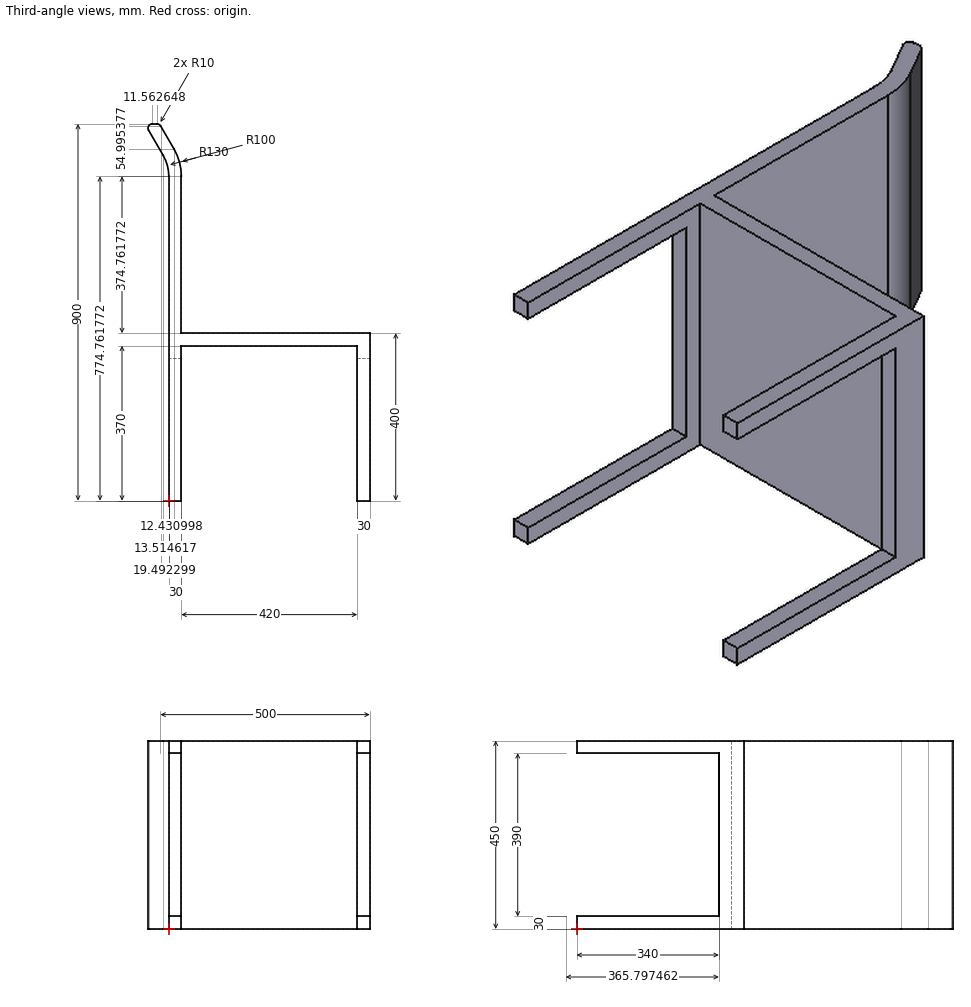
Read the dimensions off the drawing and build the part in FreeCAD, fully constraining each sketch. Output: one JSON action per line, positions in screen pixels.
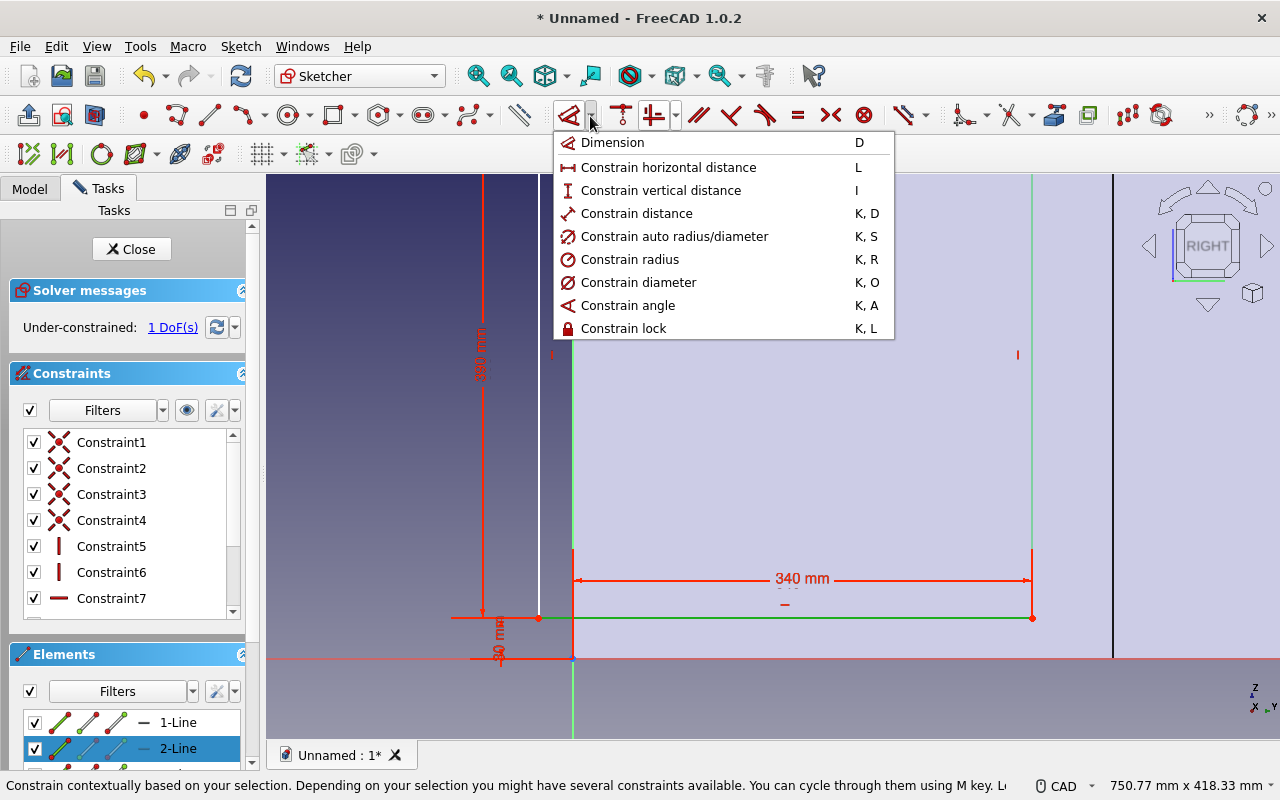
{"action": "left_click", "coordinate": [724, 168]}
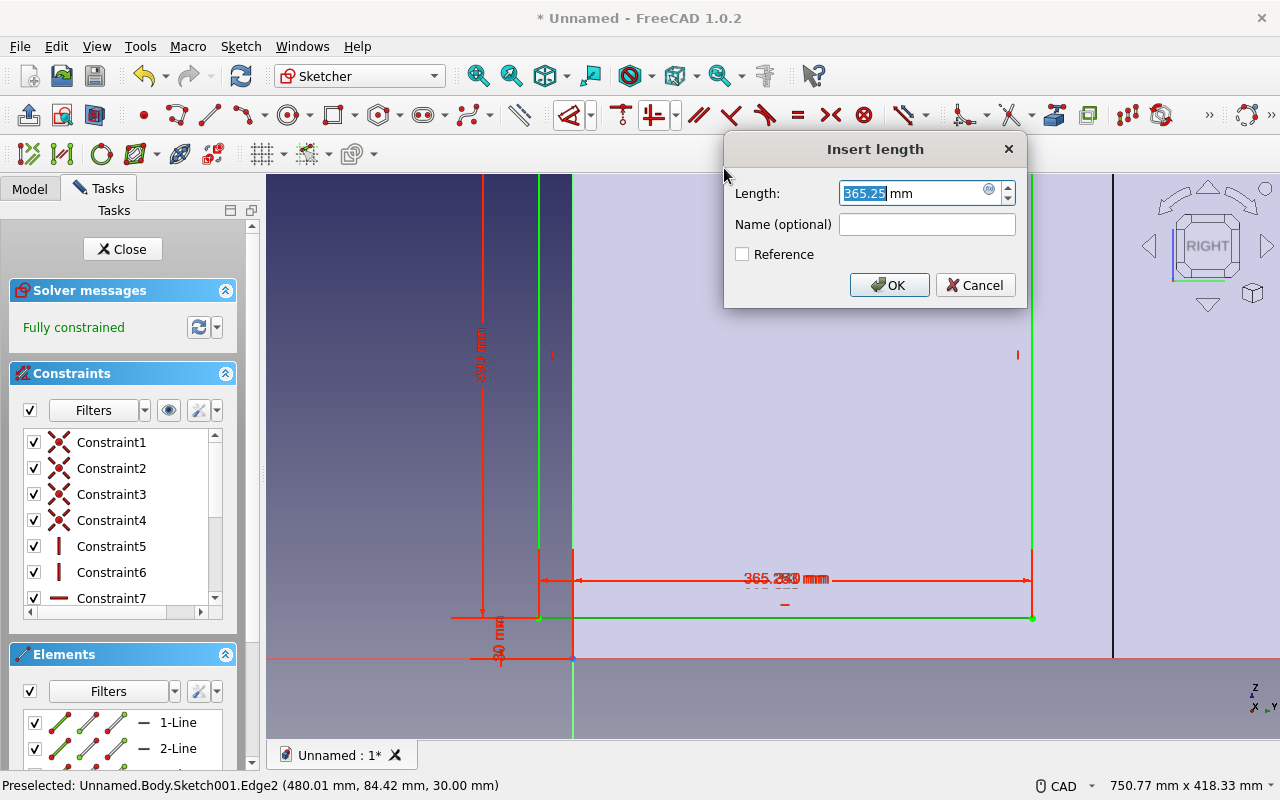
{"action": "type", "text": "365.797462"}
{"action": "key", "text": "Return"}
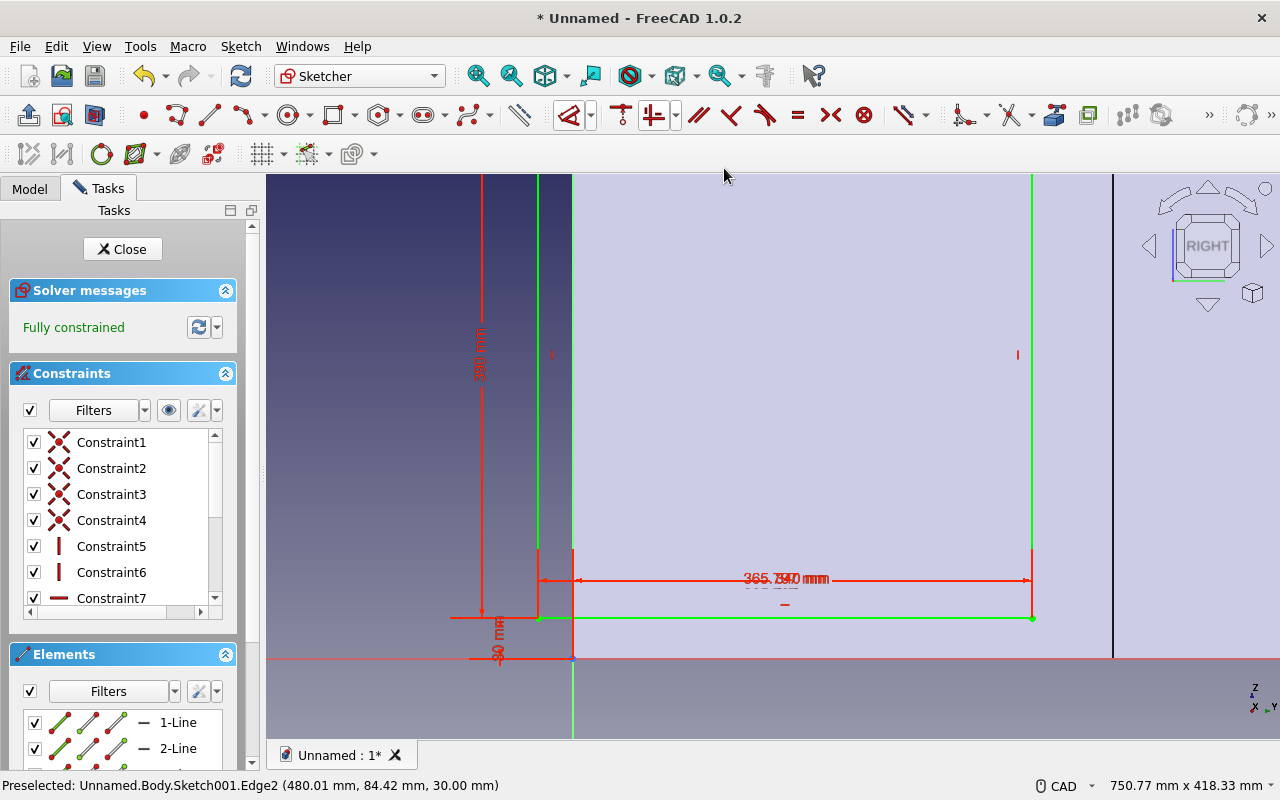
{"action": "left_click", "coordinate": [123, 249]}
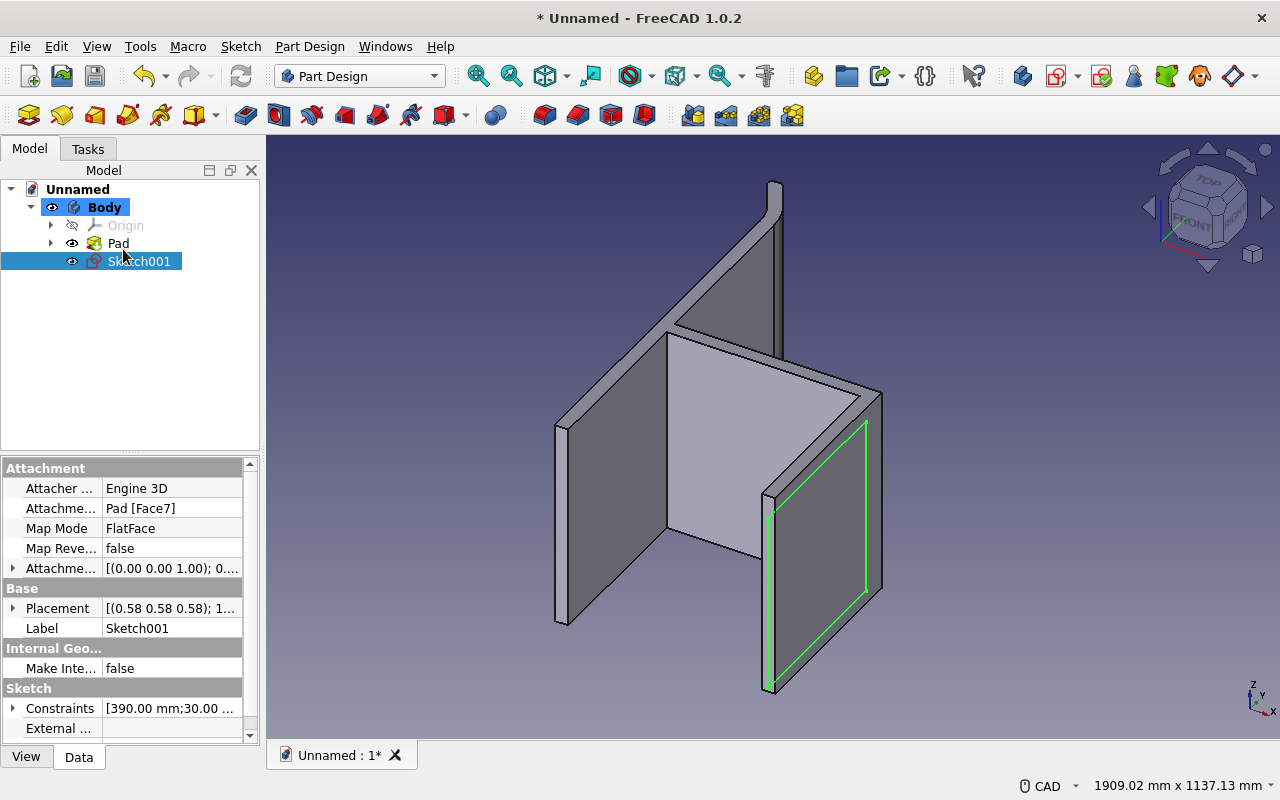
{"action": "left_click", "coordinate": [246, 116]}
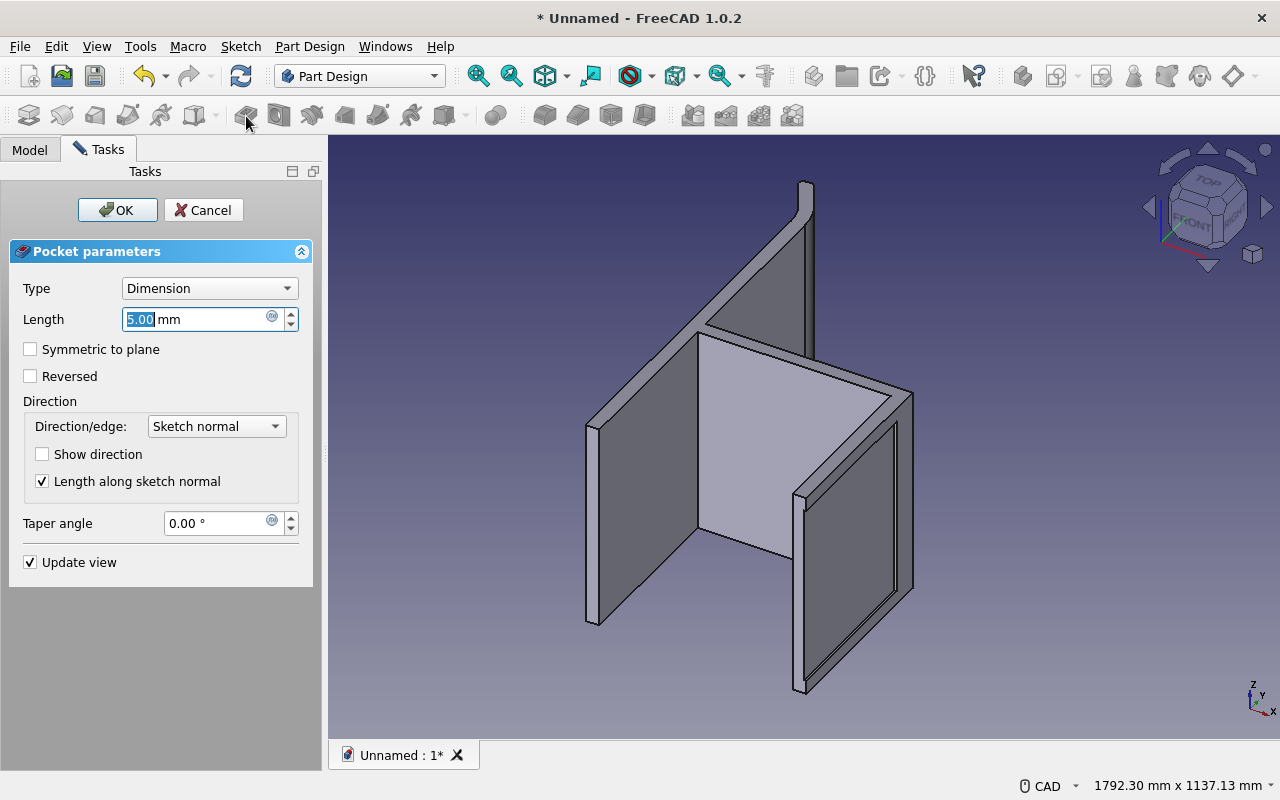
{"action": "type", "text": "500"}
{"action": "key", "text": "Tab"}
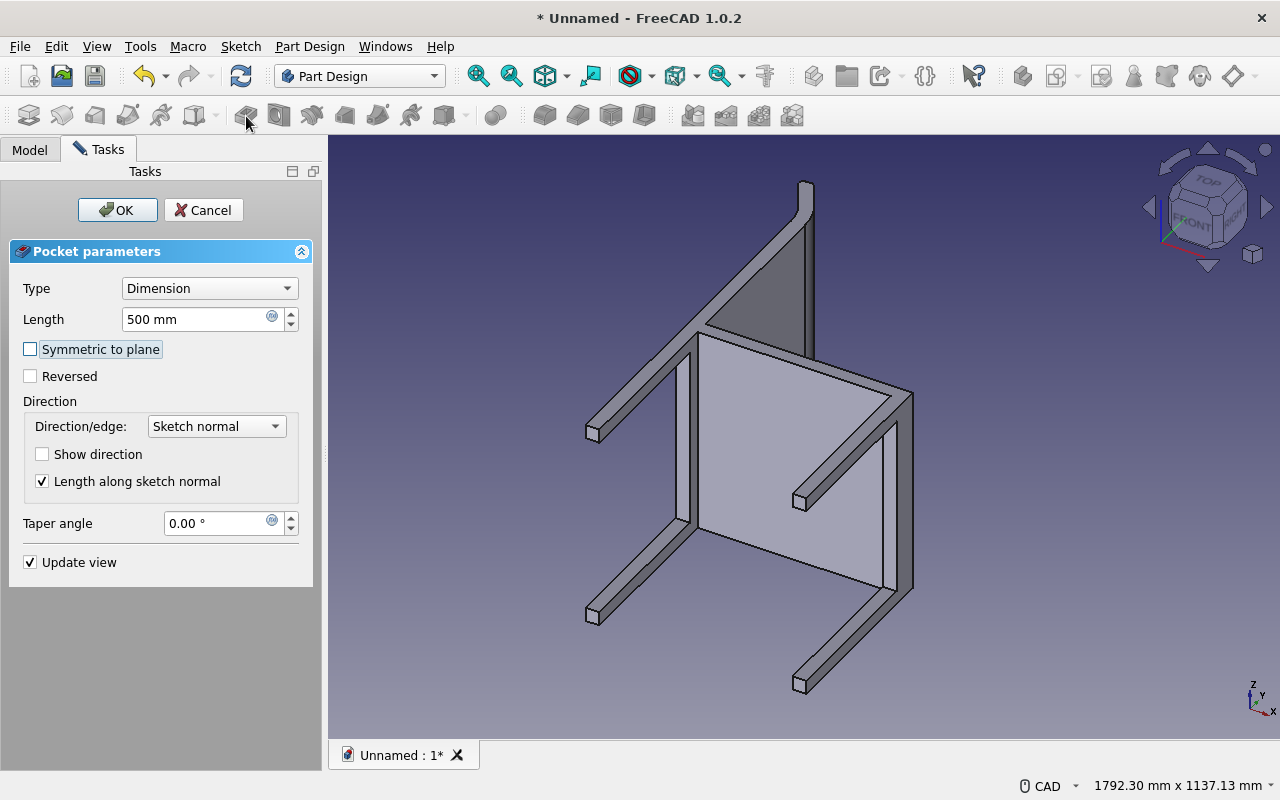
{"action": "left_click", "coordinate": [118, 210]}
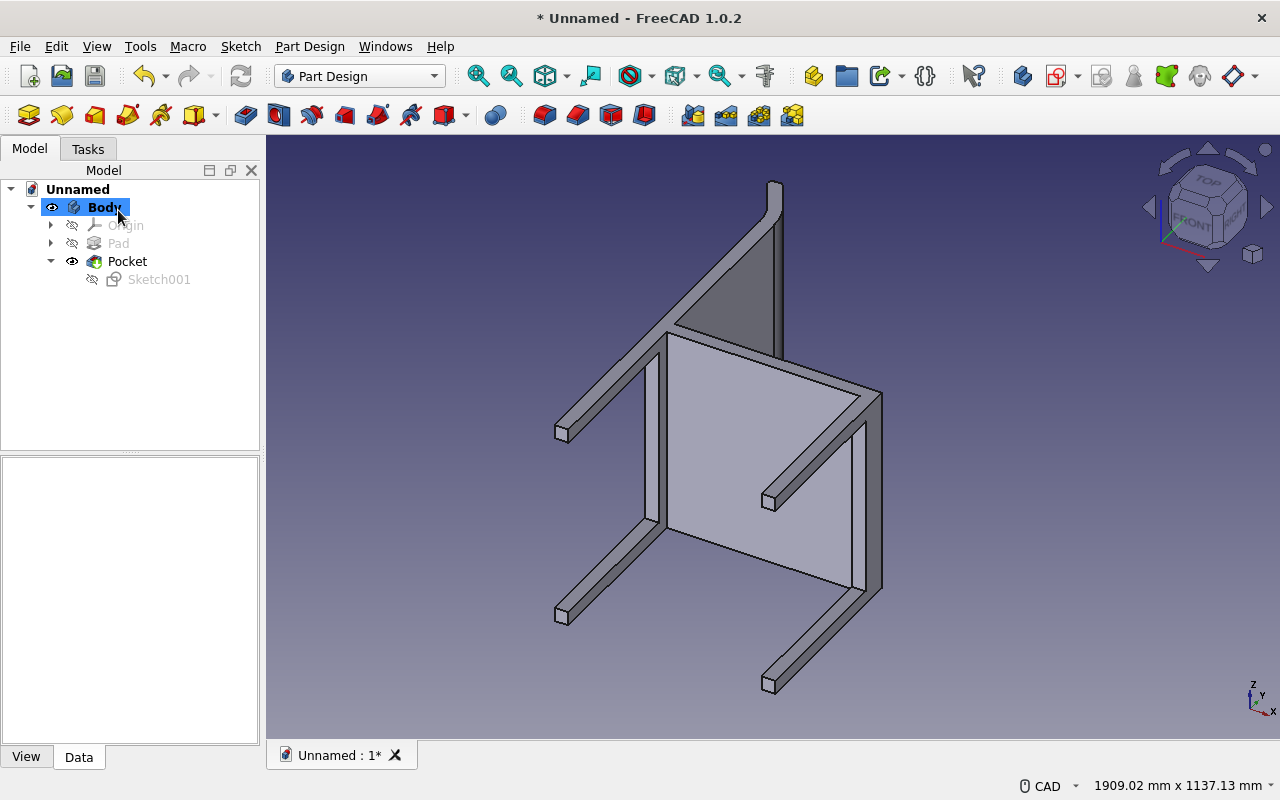
{"action": "key", "text": "0"}